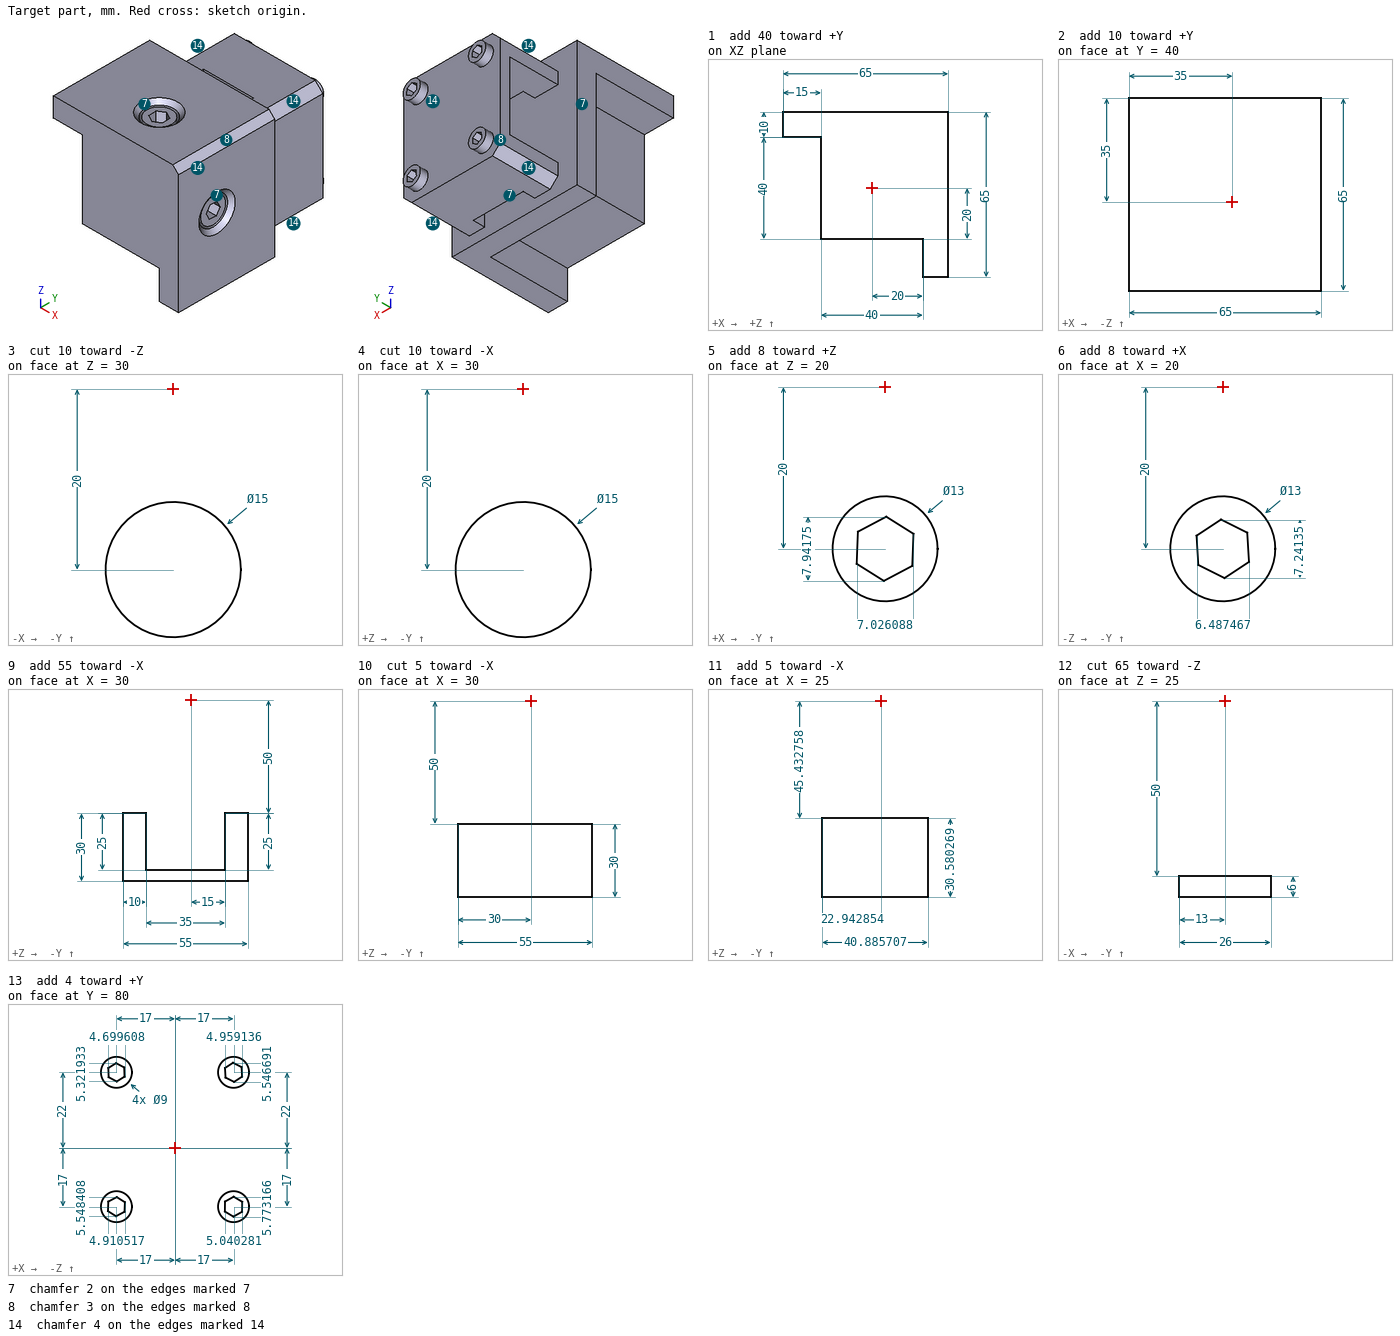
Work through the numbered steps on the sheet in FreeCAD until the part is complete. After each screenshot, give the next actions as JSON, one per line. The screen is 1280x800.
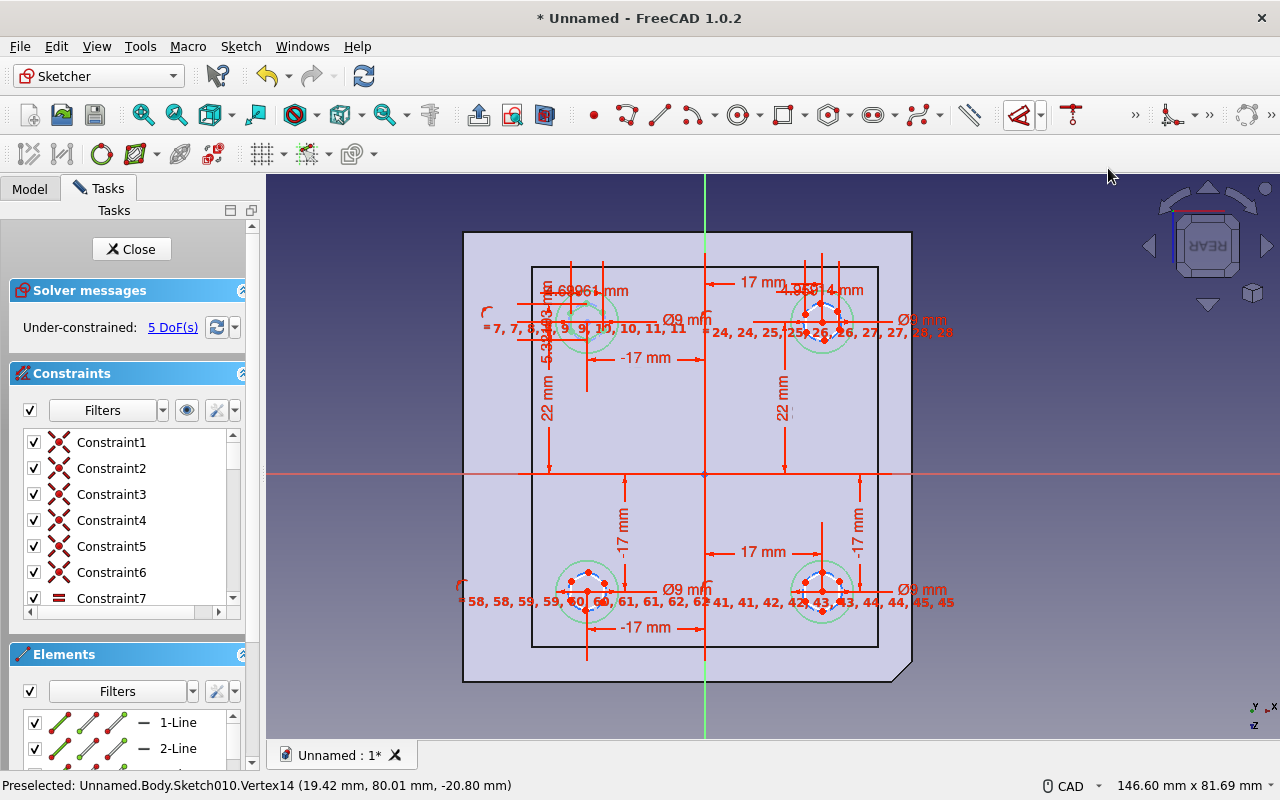
{"action": "left_click", "coordinate": [824, 341]}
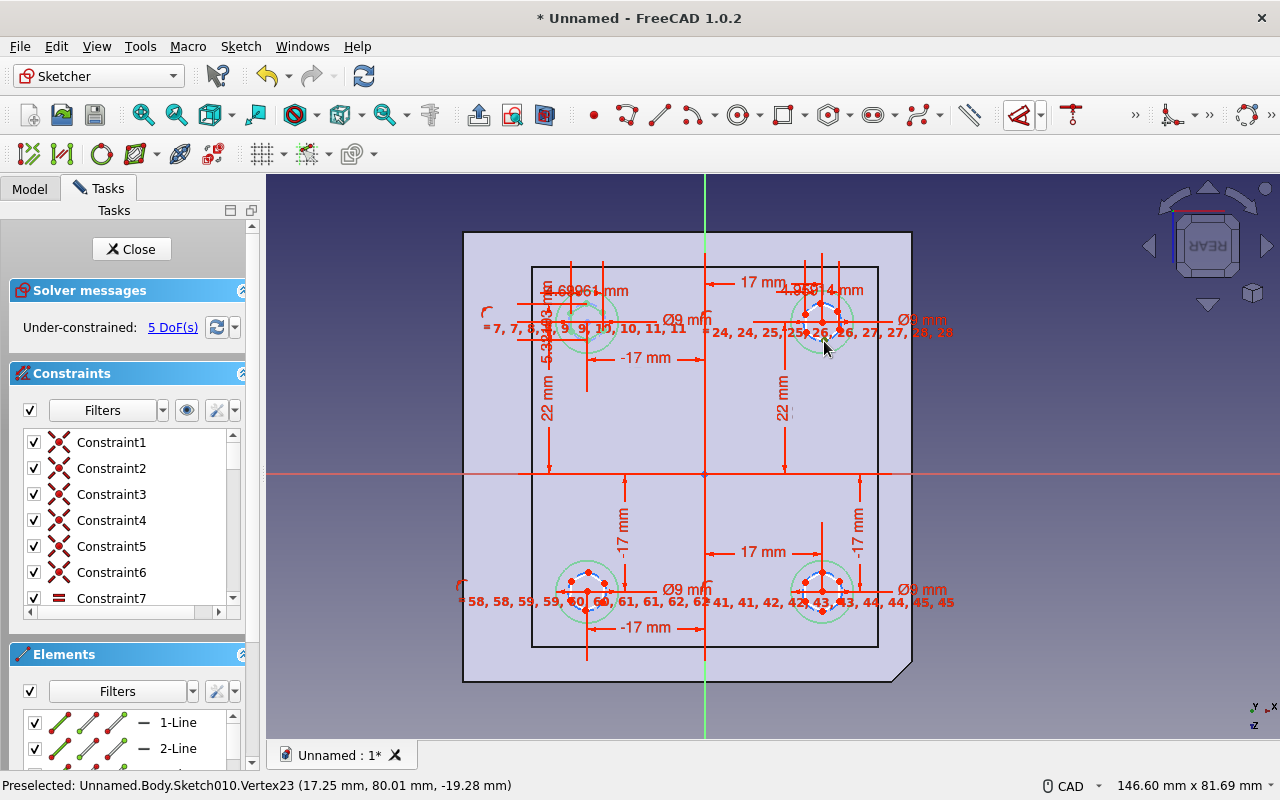
{"action": "left_click", "coordinate": [821, 303]}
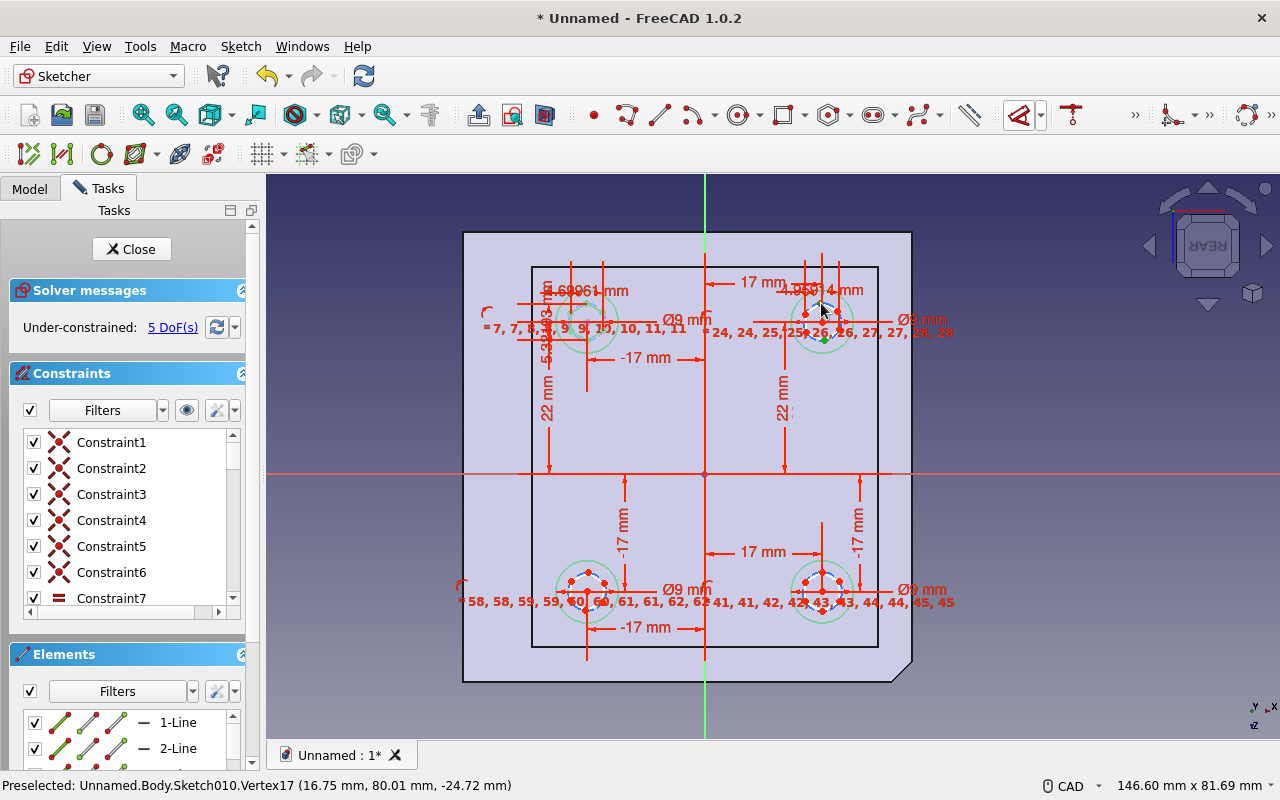
{"action": "key", "text": "i"}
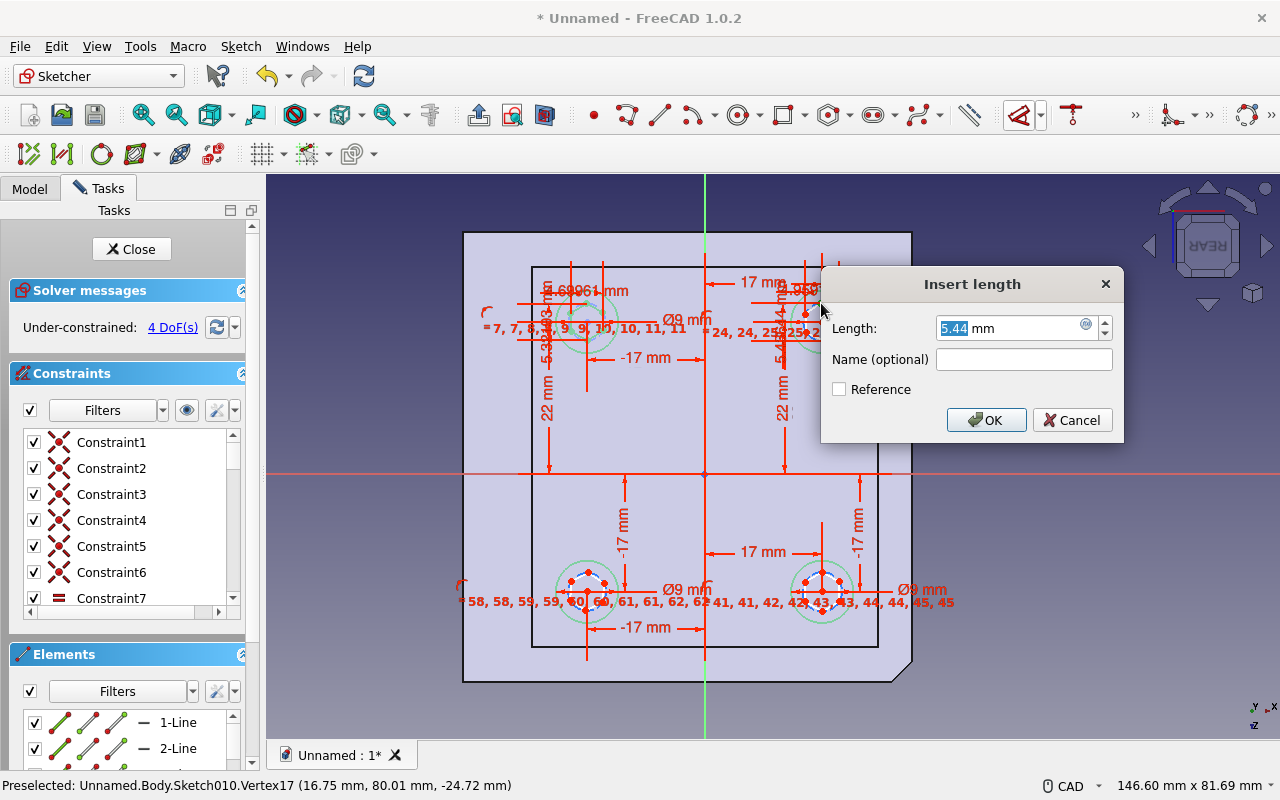
{"action": "type", "text": "5.546691"}
{"action": "key", "text": "Return"}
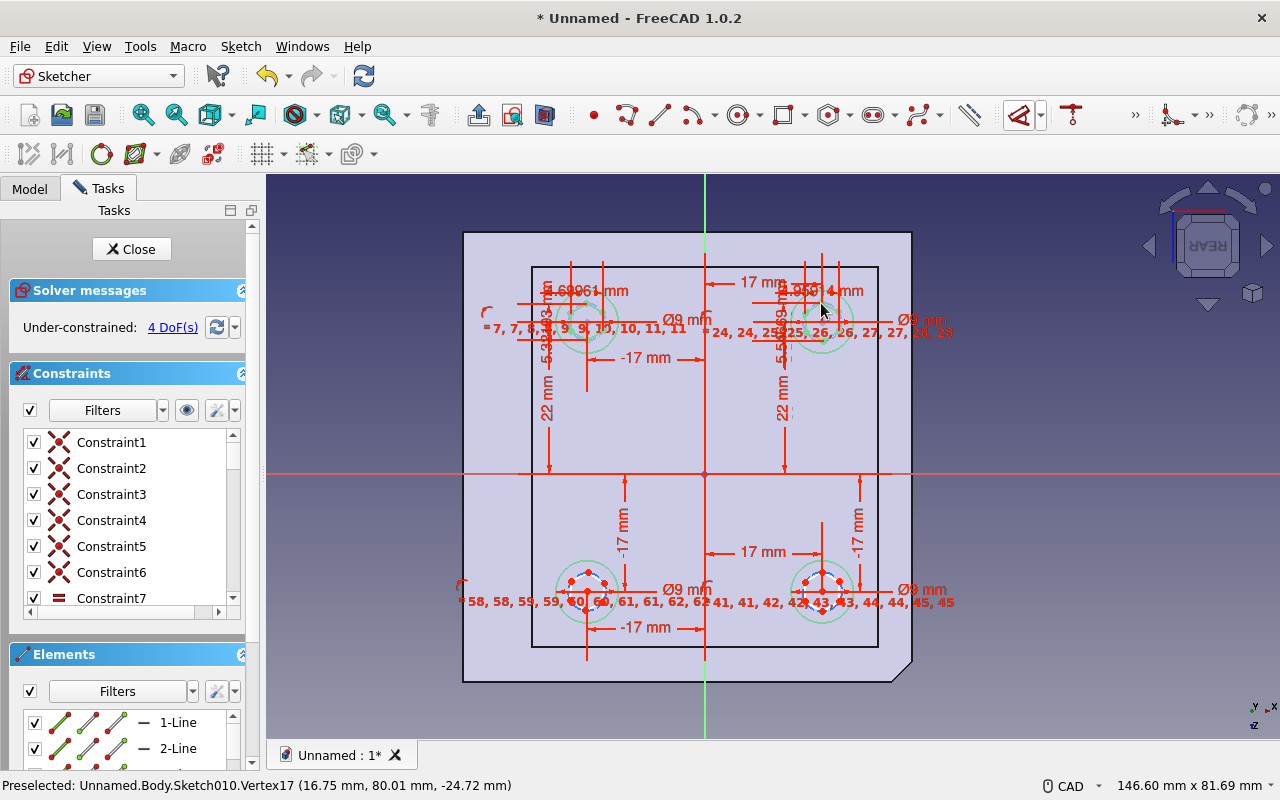
{"action": "left_click", "coordinate": [805, 602]}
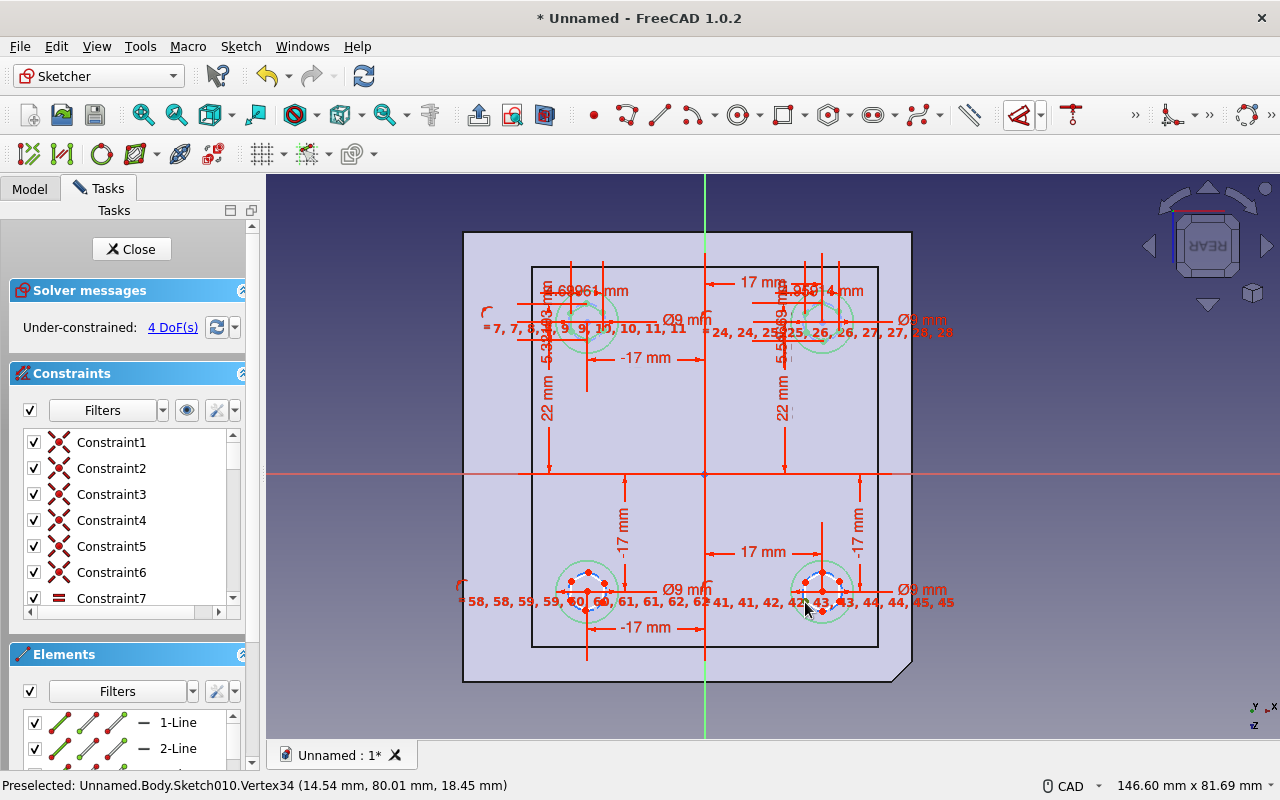
{"action": "left_click", "coordinate": [839, 582]}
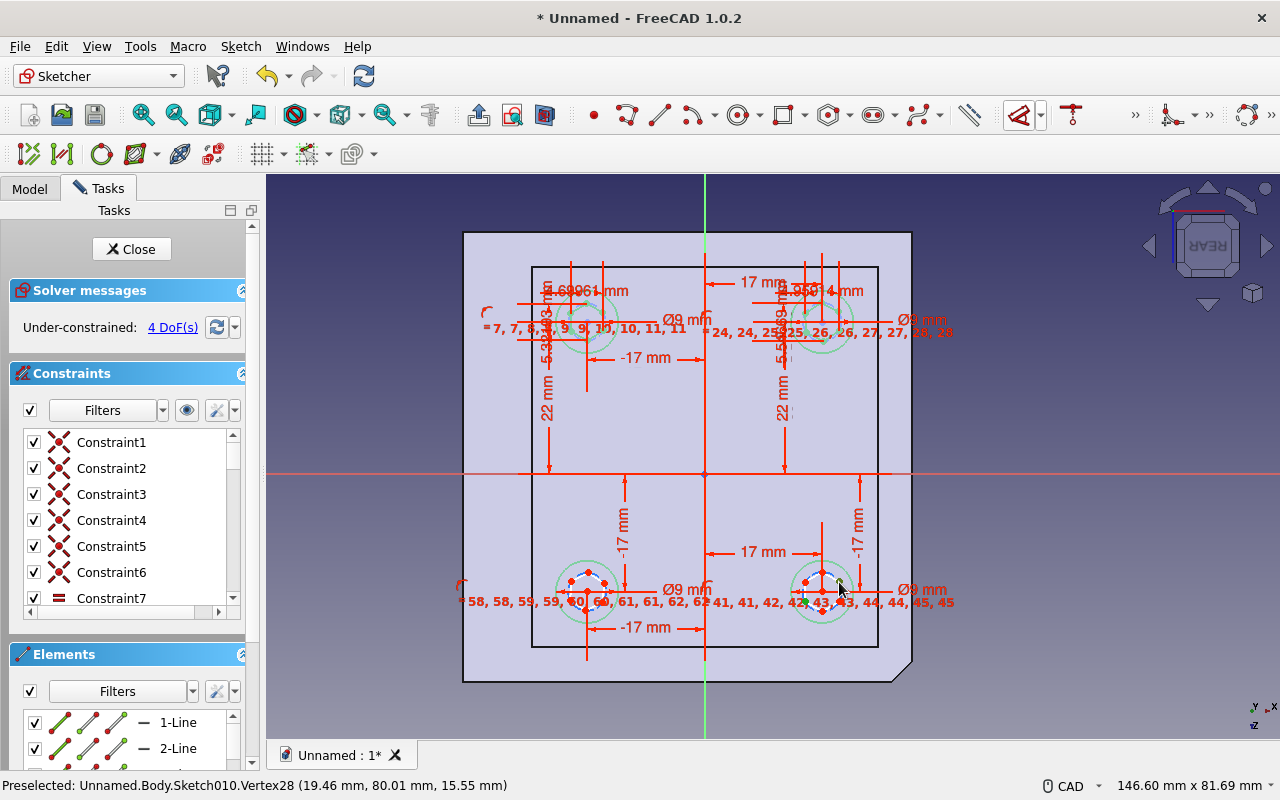
{"action": "key", "text": "l"}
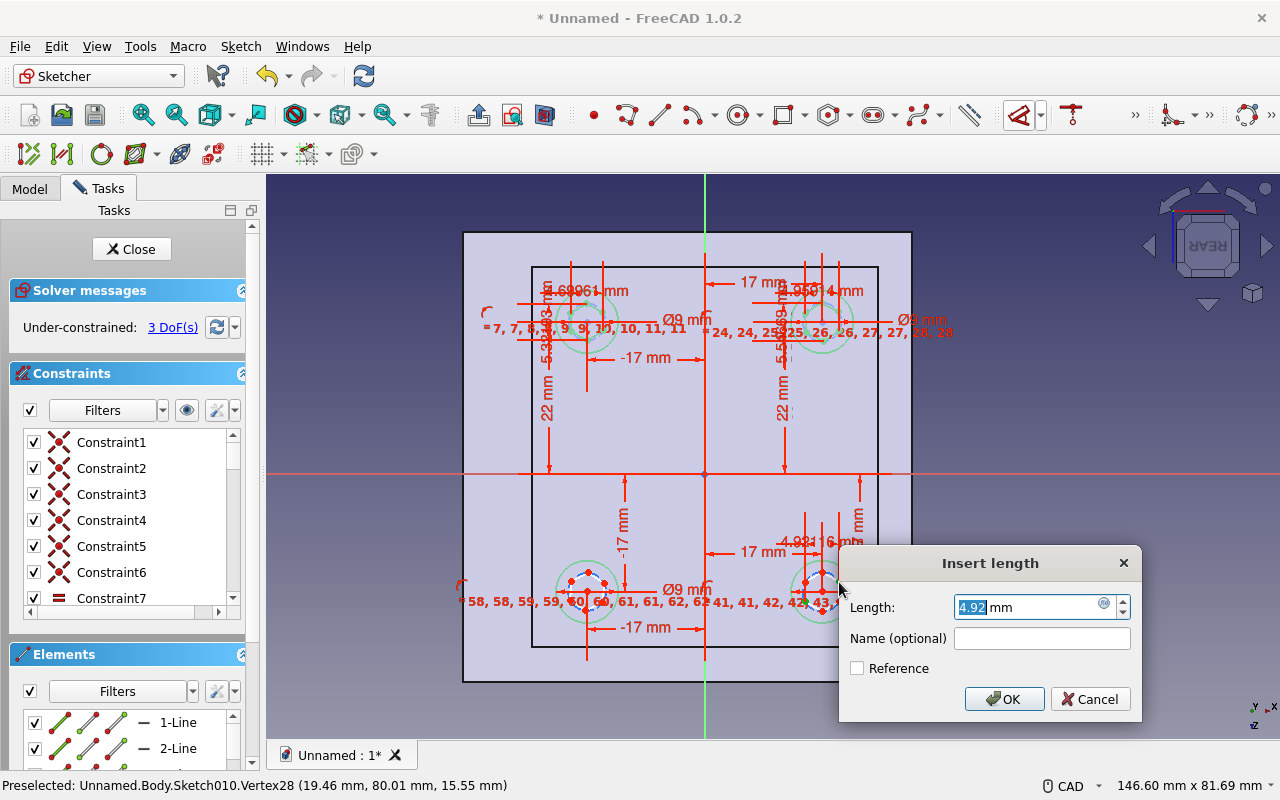
{"action": "type", "text": "5.040281"}
{"action": "key", "text": "Return"}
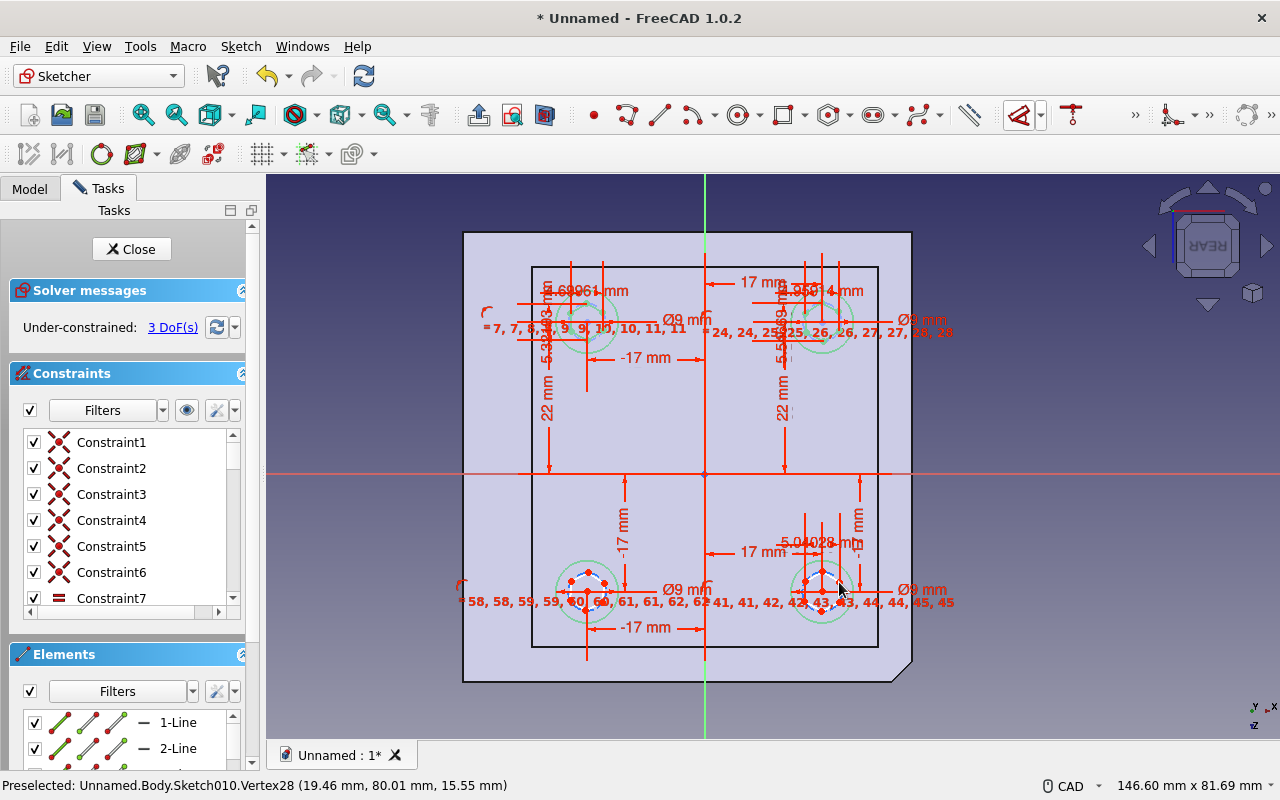
{"action": "left_click", "coordinate": [822, 612]}